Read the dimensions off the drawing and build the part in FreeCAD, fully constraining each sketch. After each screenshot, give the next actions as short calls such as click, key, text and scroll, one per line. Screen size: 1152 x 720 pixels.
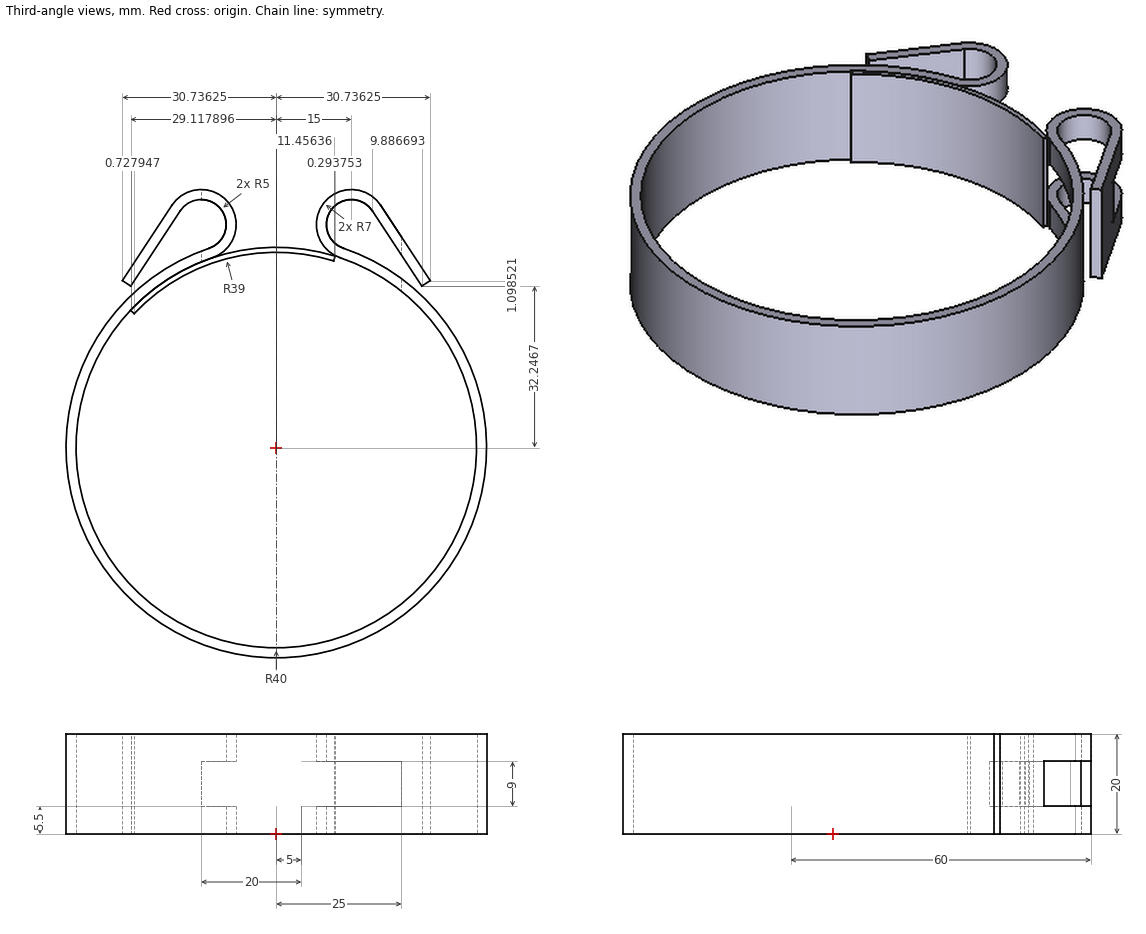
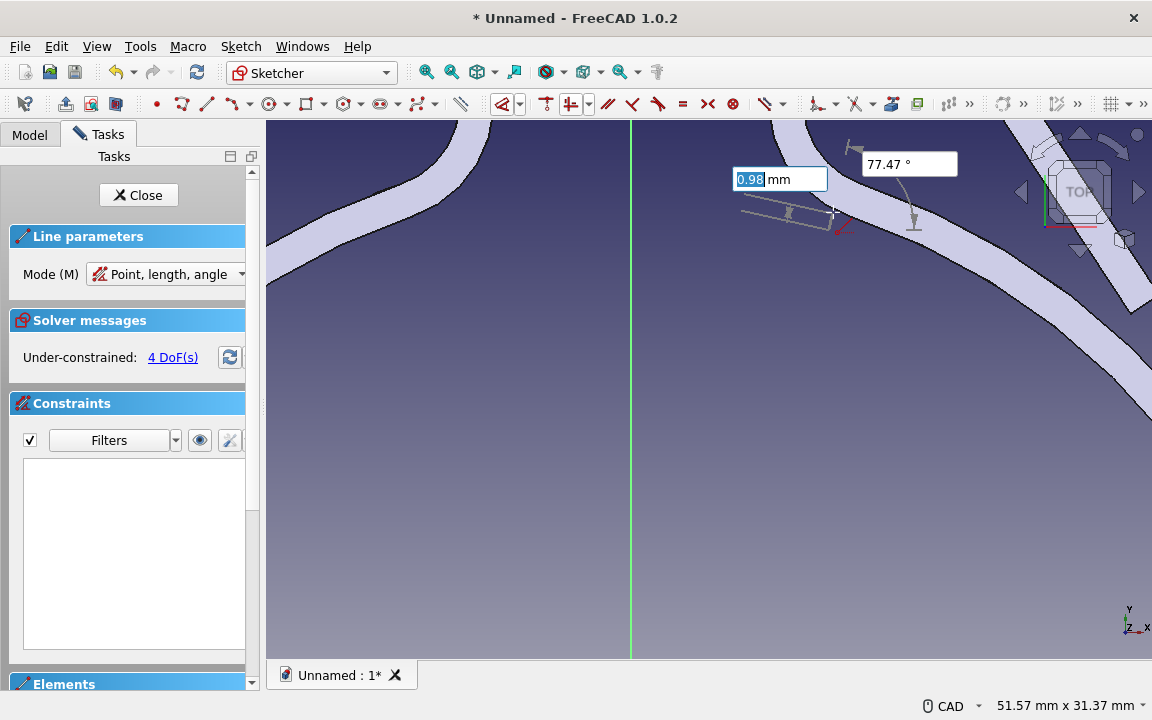
click(833, 211)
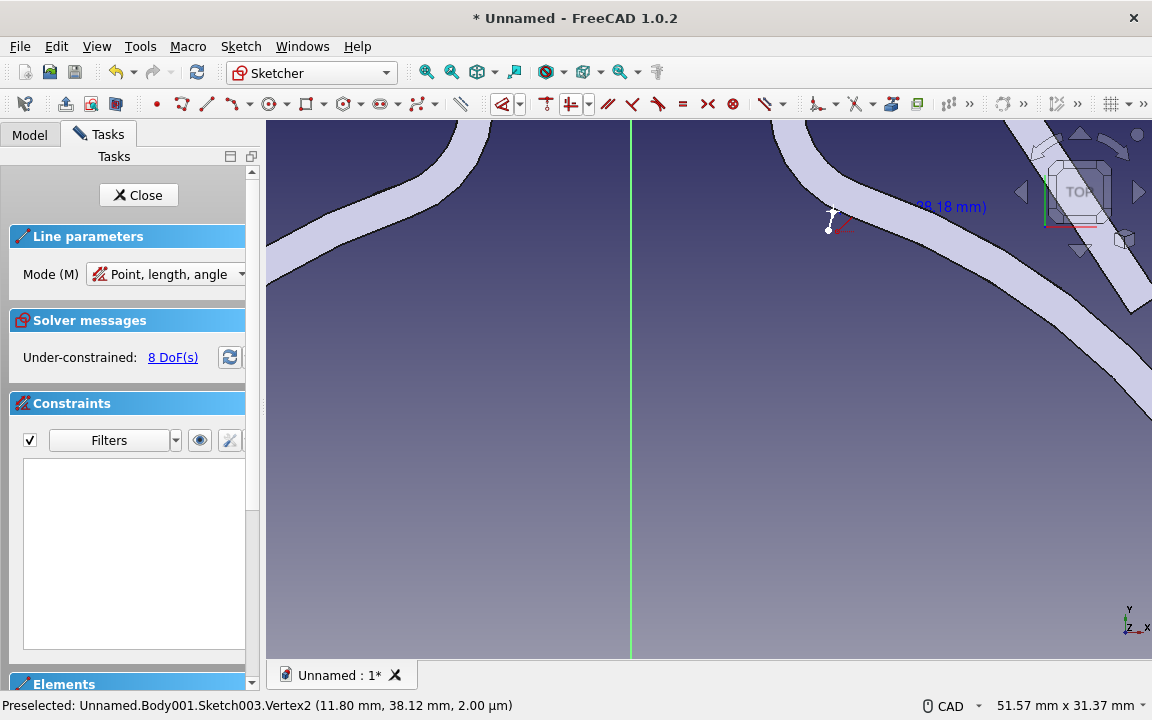
click(232, 104)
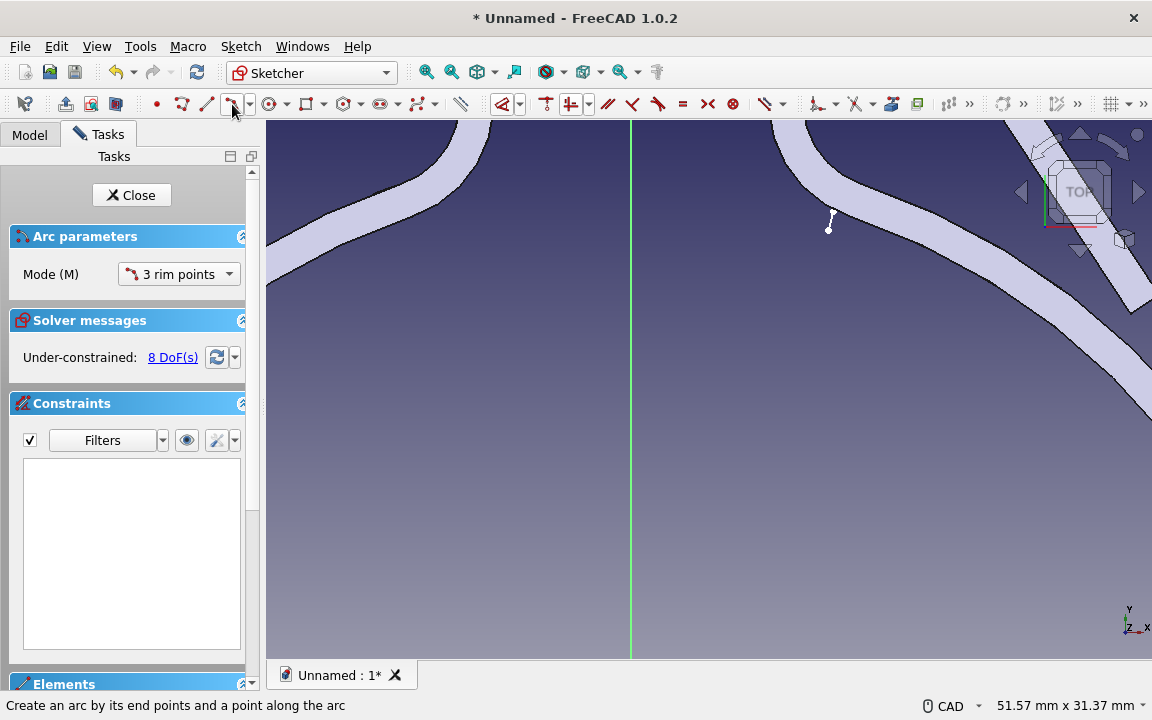
scroll(833, 212, down, 3)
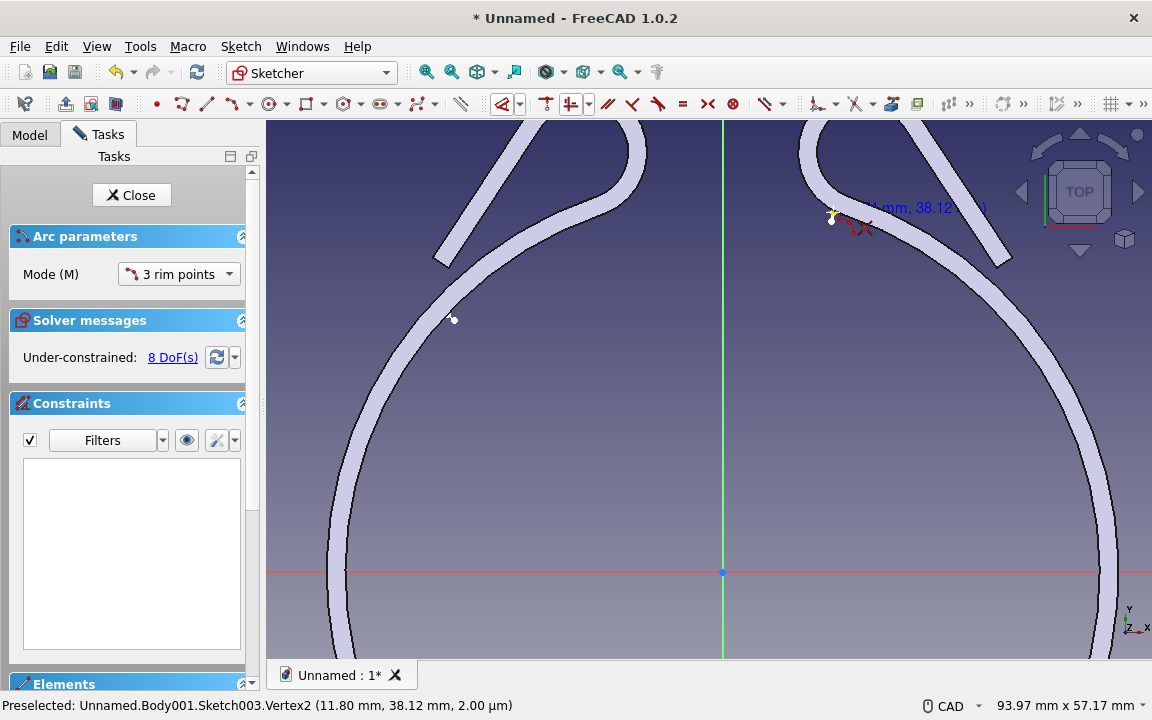
scroll(455, 320, up, 7)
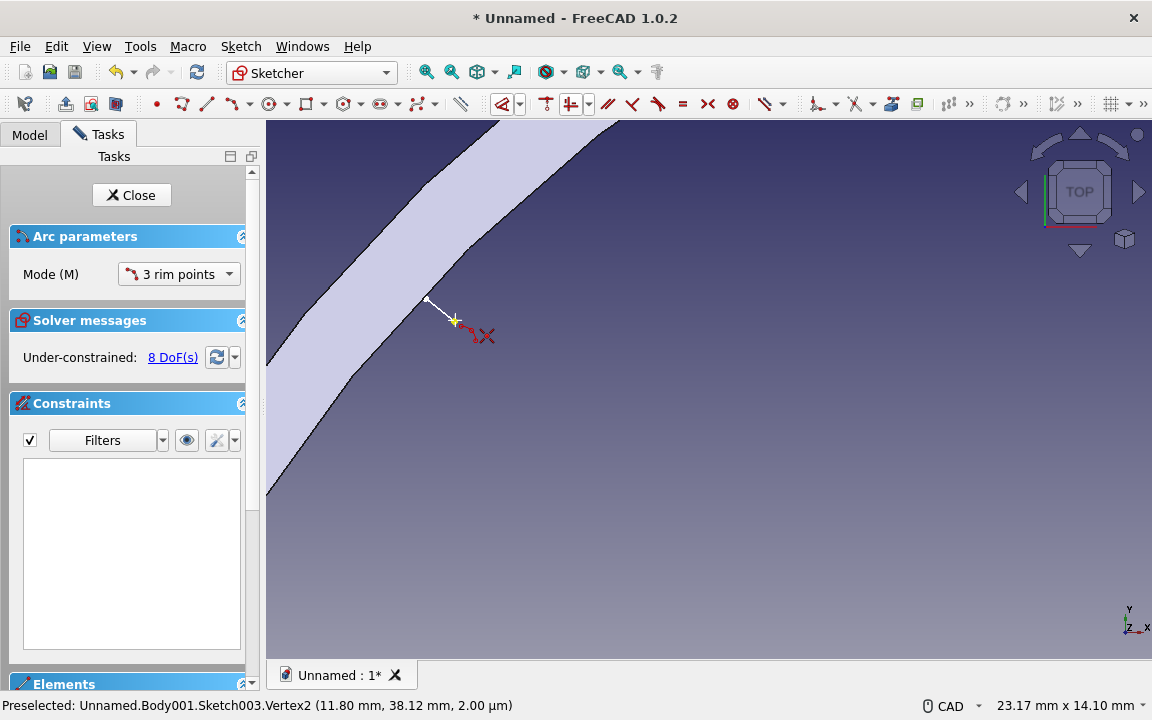
click(454, 321)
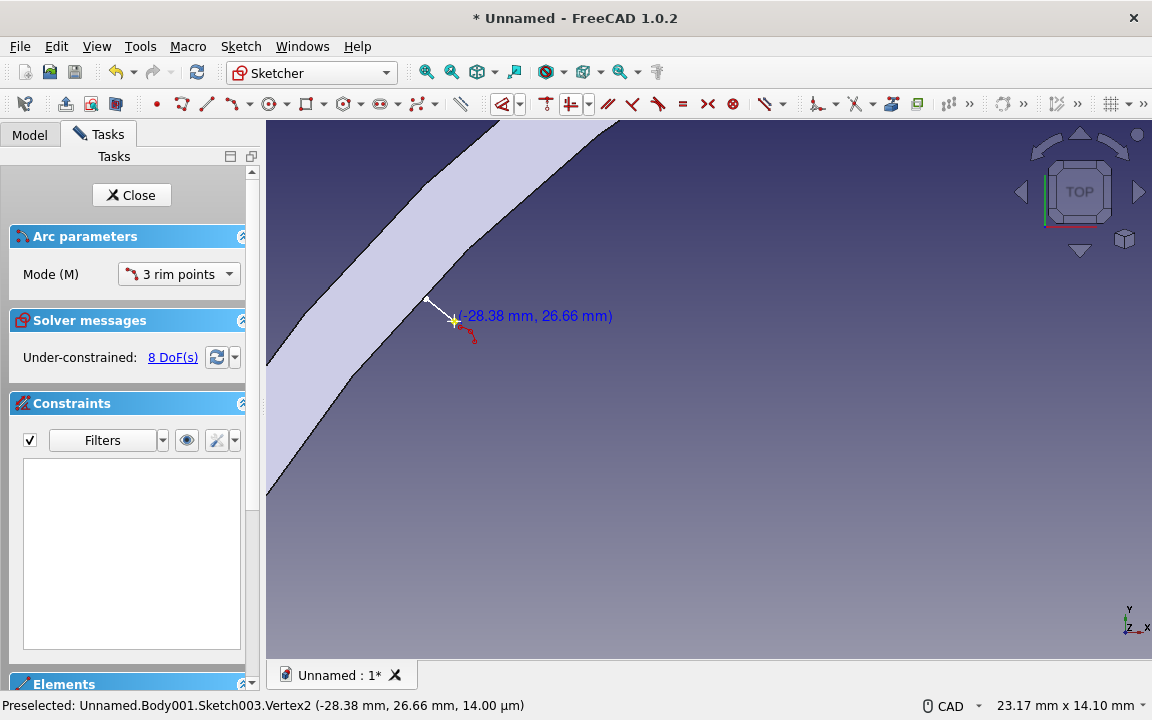
scroll(455, 320, down, 7)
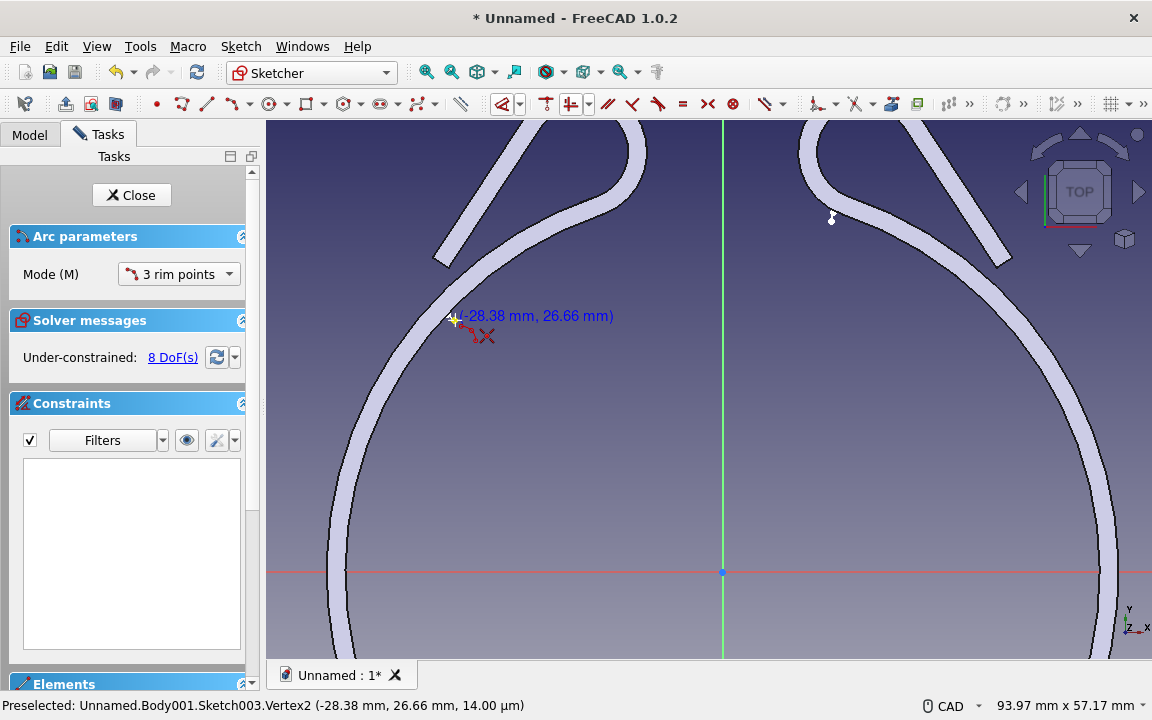
scroll(831, 221, up, 7)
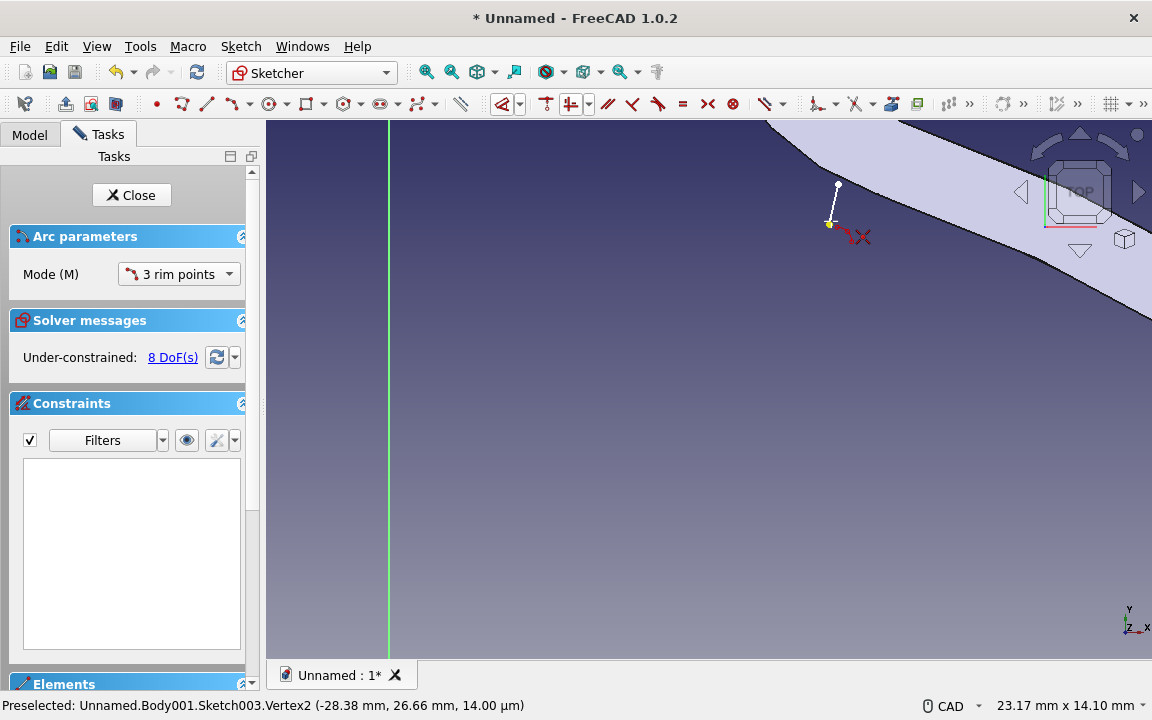
click(829, 224)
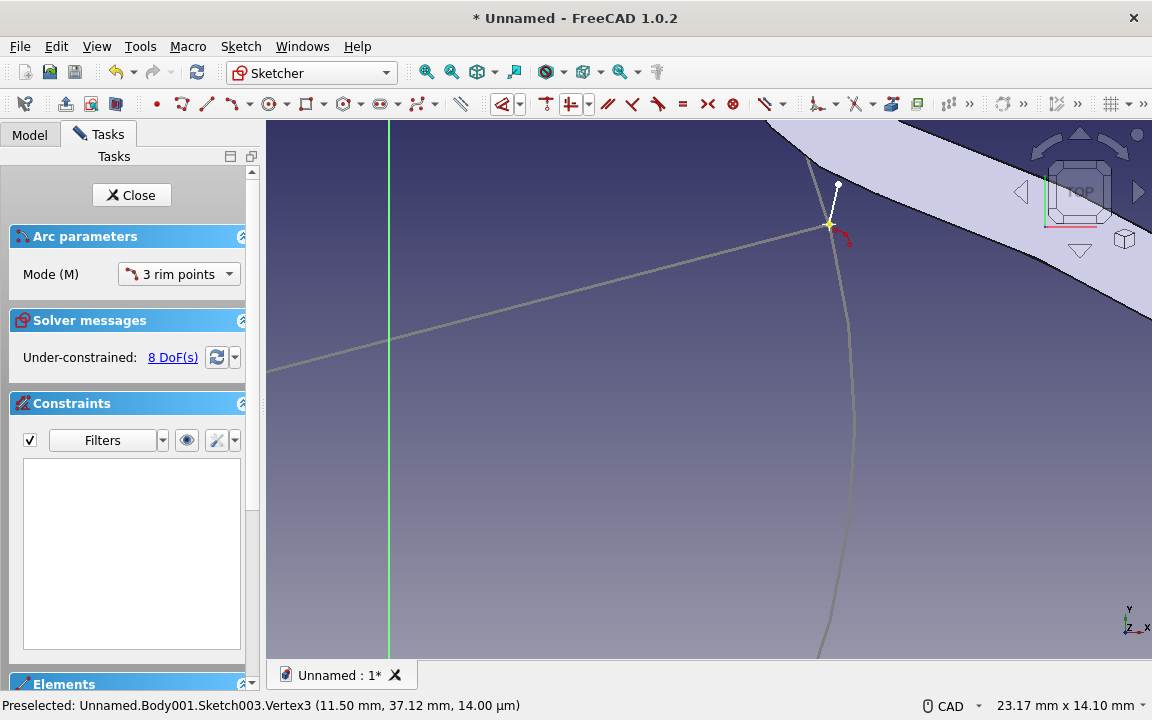
scroll(831, 221, down, 7)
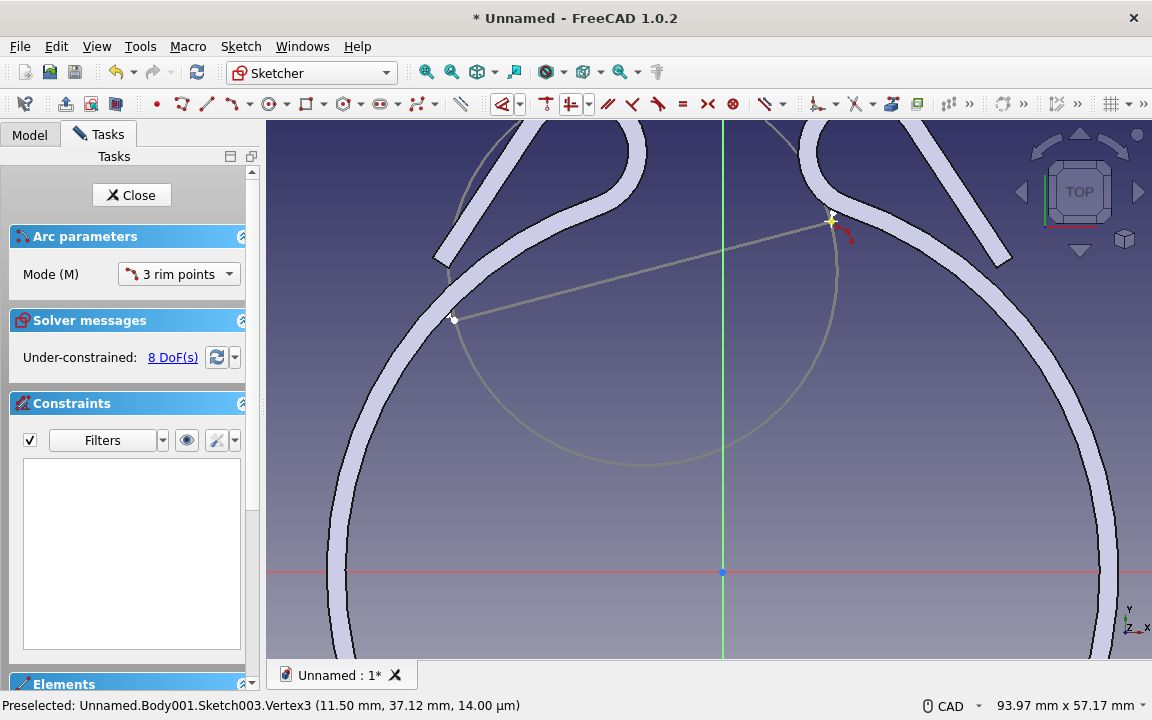
click(629, 217)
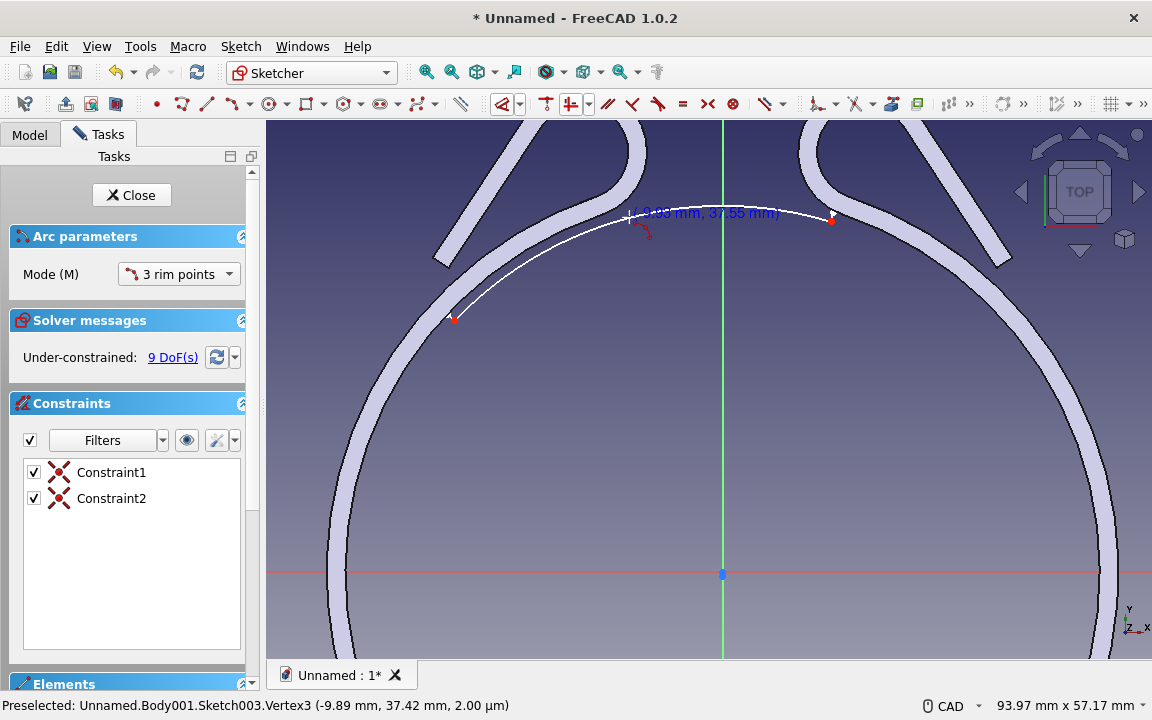
scroll(833, 212, up, 7)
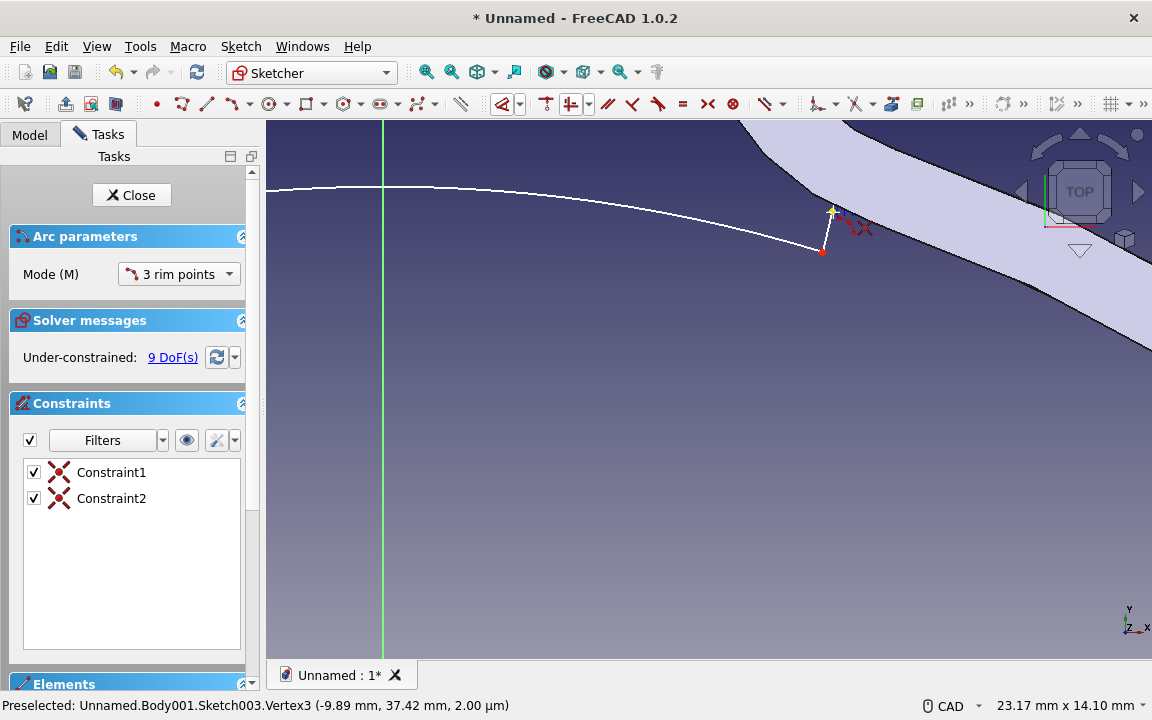
click(832, 212)